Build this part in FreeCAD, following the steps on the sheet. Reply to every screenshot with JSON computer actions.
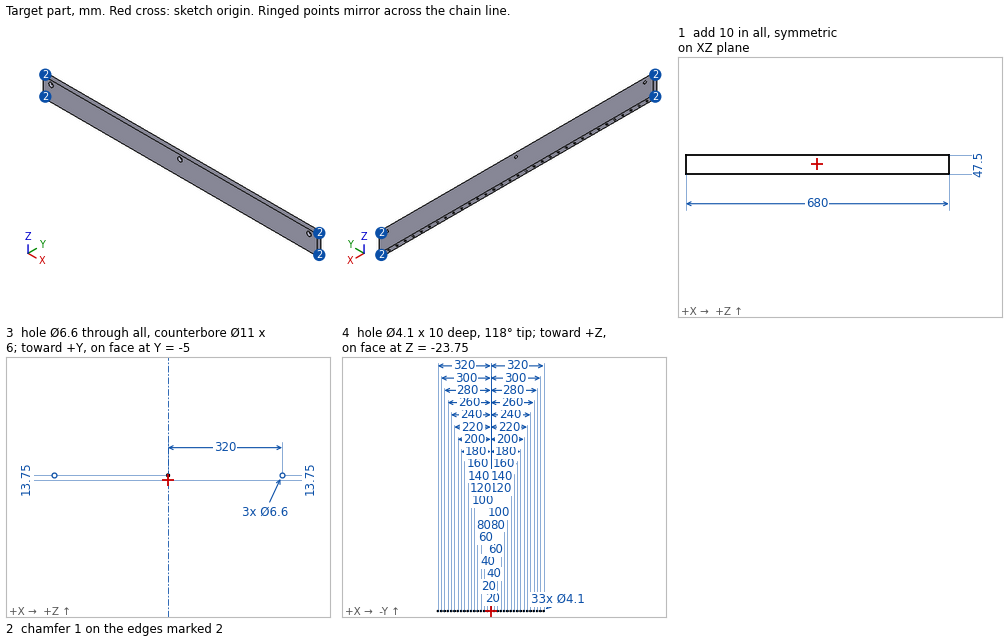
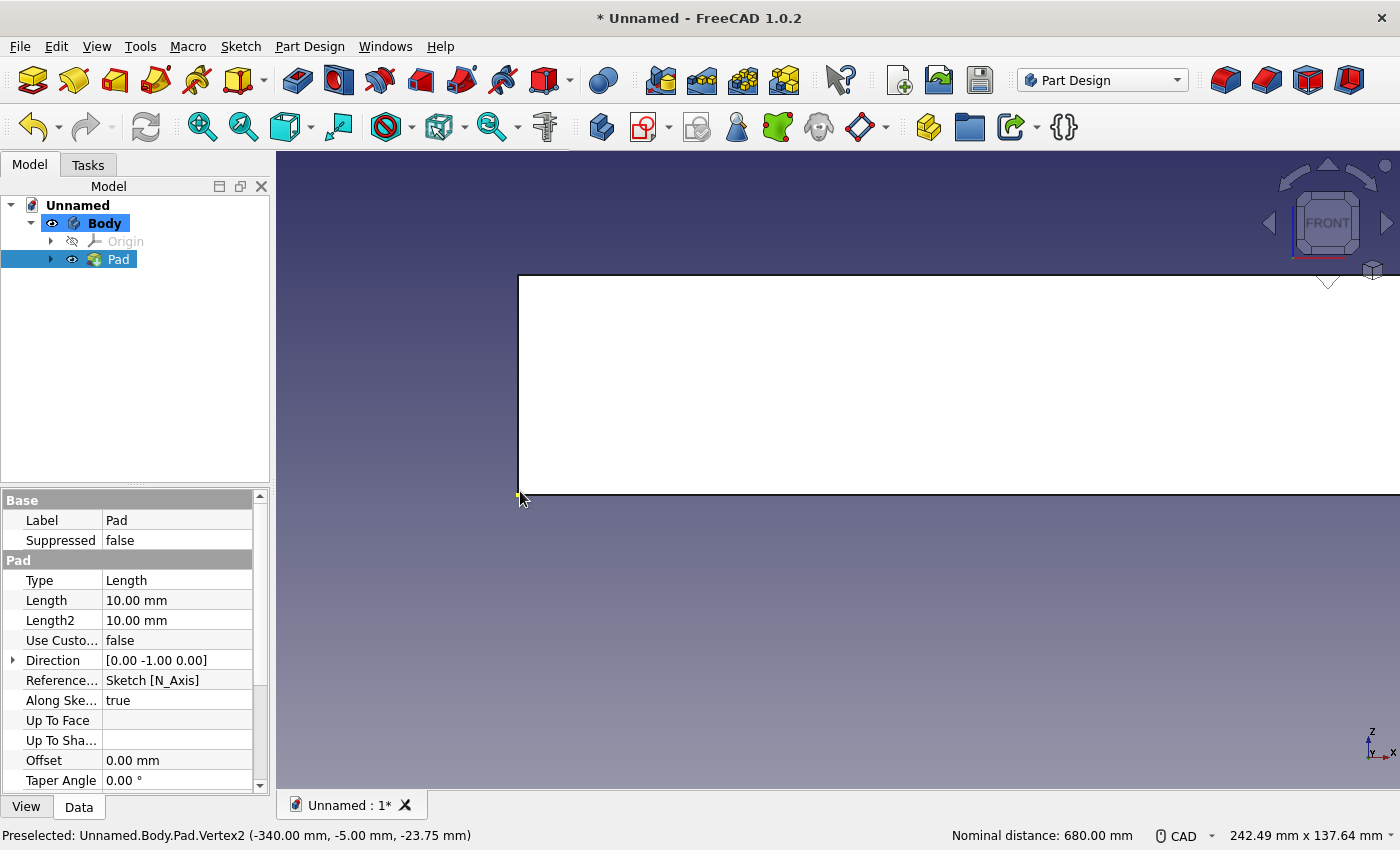
{"action": "left_click", "coordinate": [203, 128]}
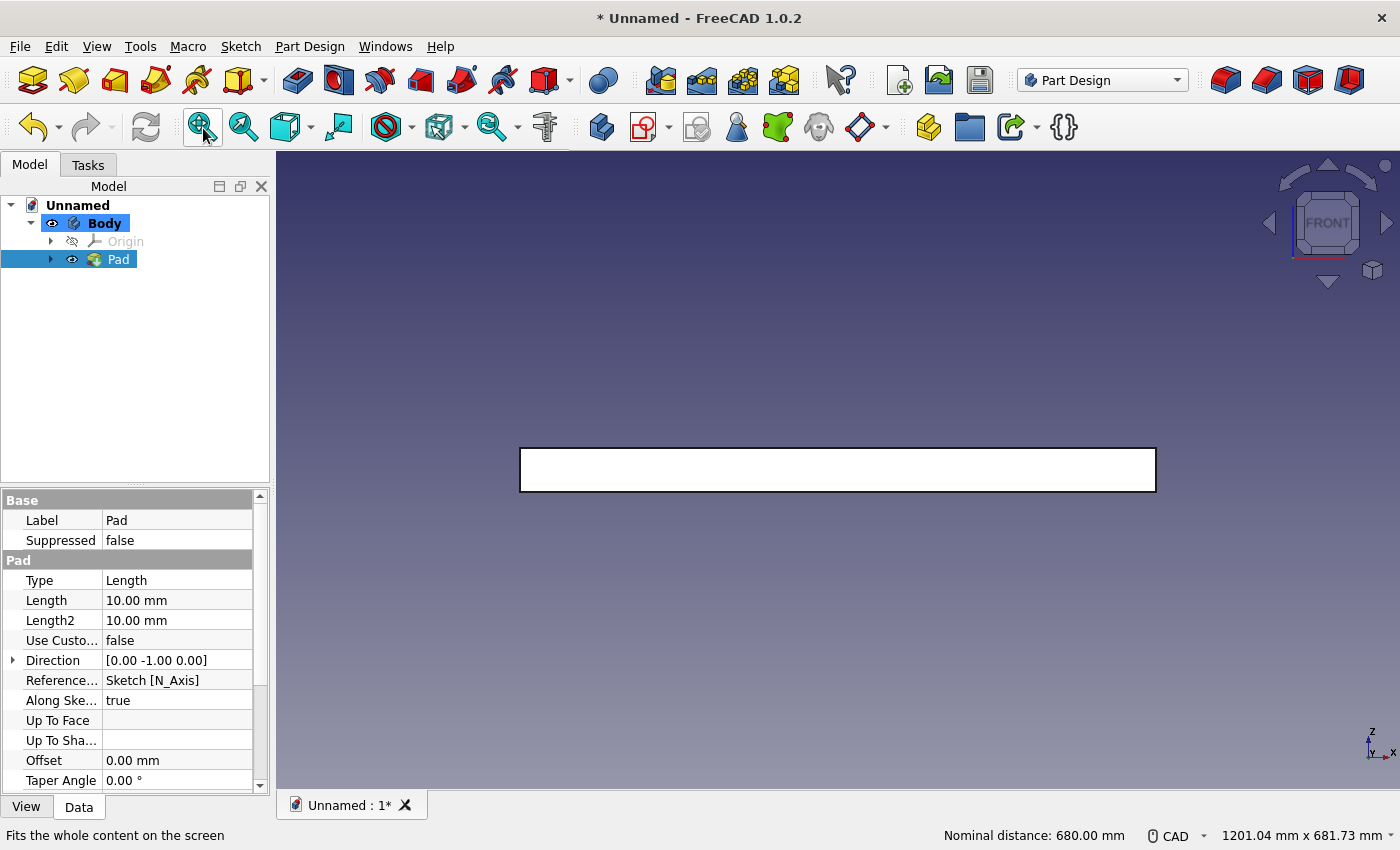
{"action": "key", "text": "3"}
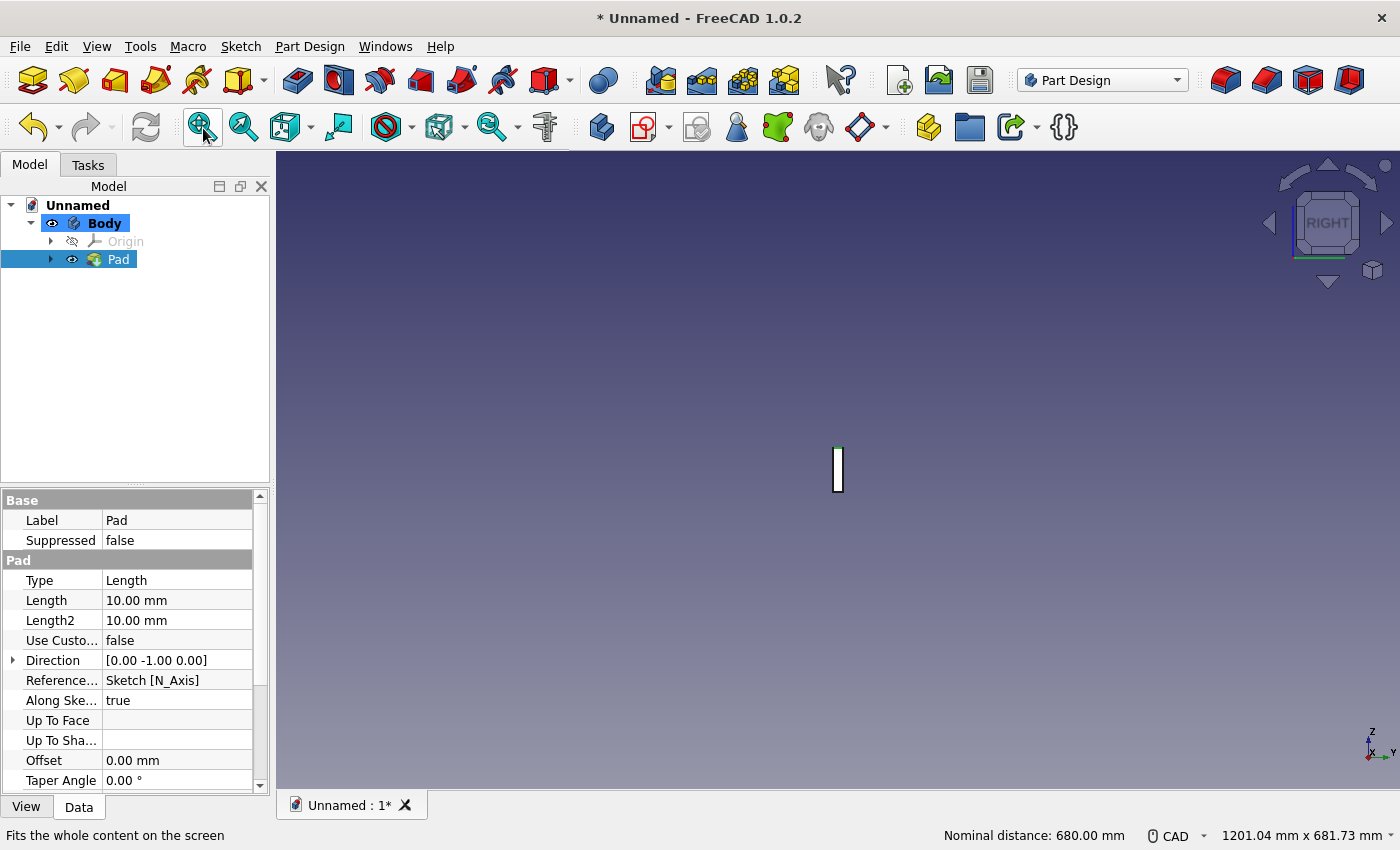
{"action": "left_click", "coordinate": [203, 128]}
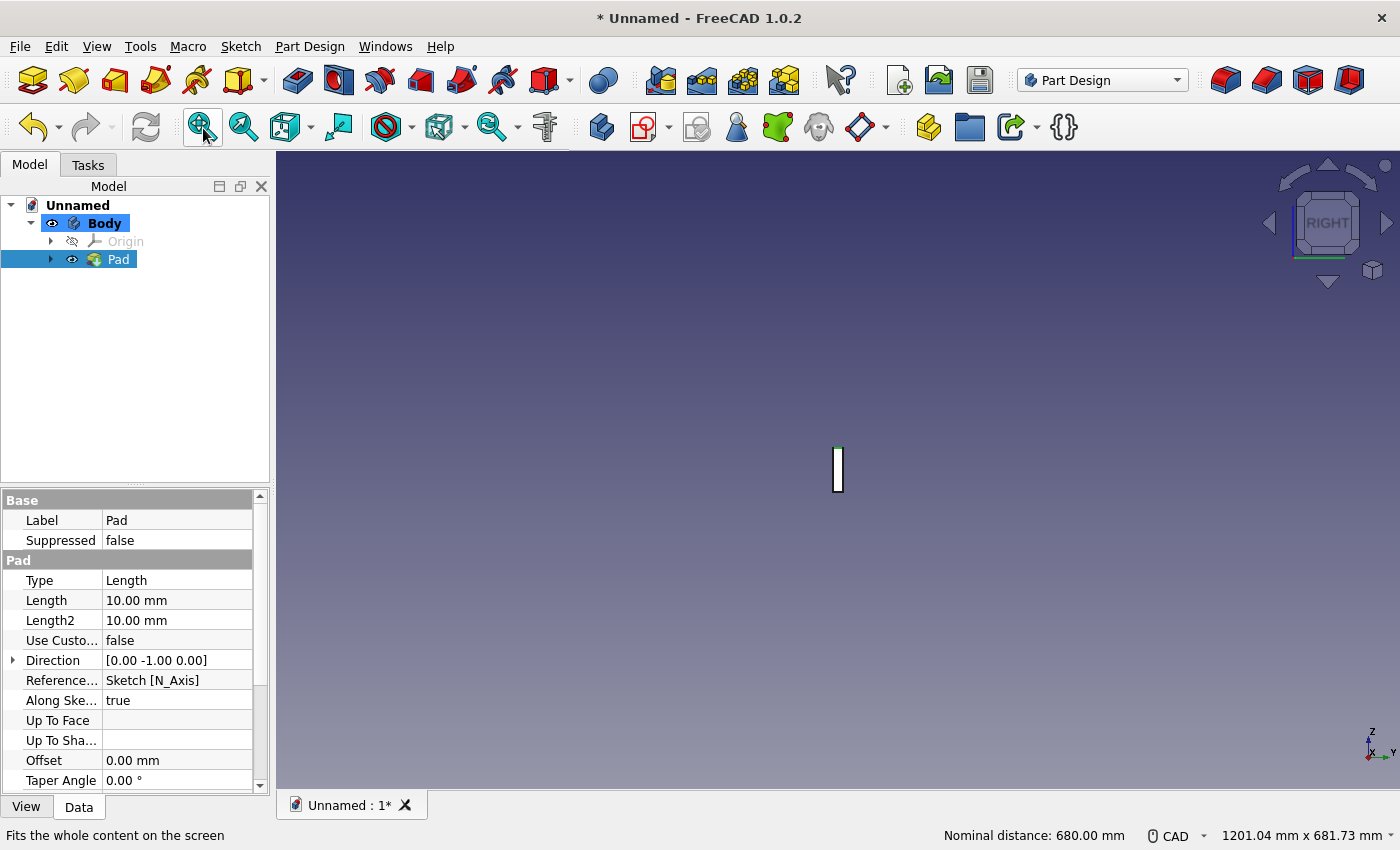
{"action": "scroll", "coordinate": [838, 491], "scroll_direction": "up", "scroll_amount": 8}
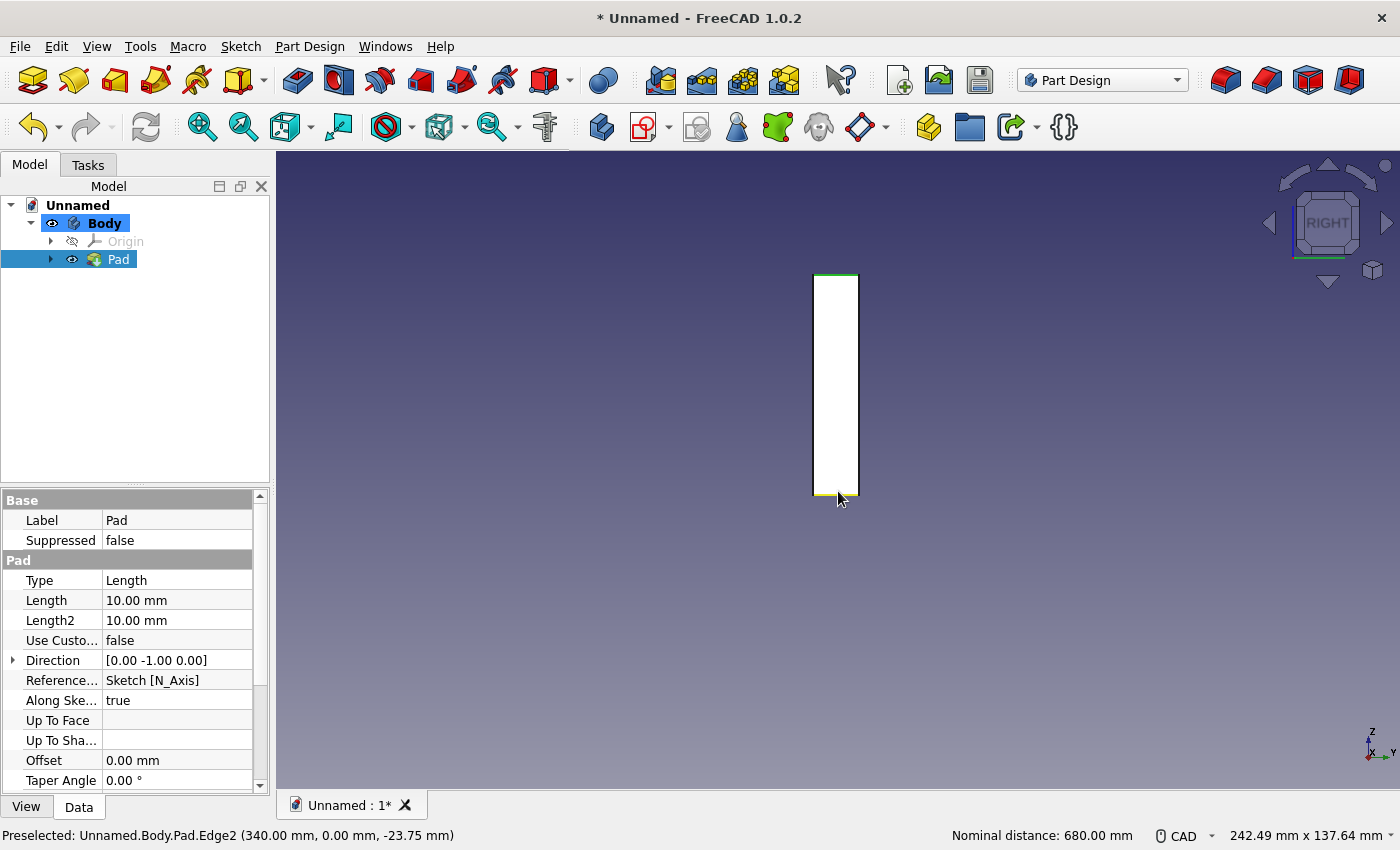
{"action": "left_click", "coordinate": [836, 494], "text": "ctrl"}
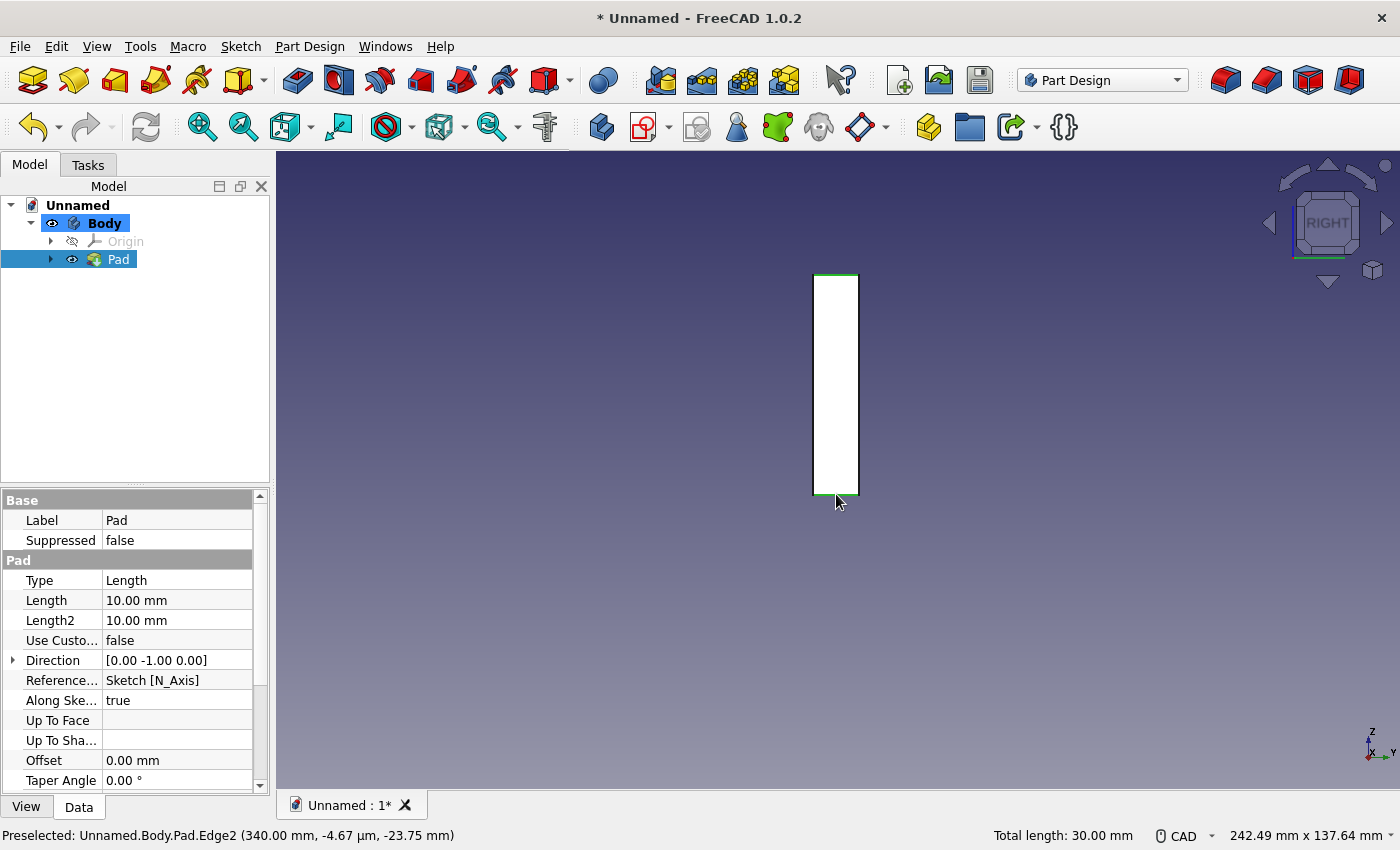
{"action": "left_click", "coordinate": [203, 128]}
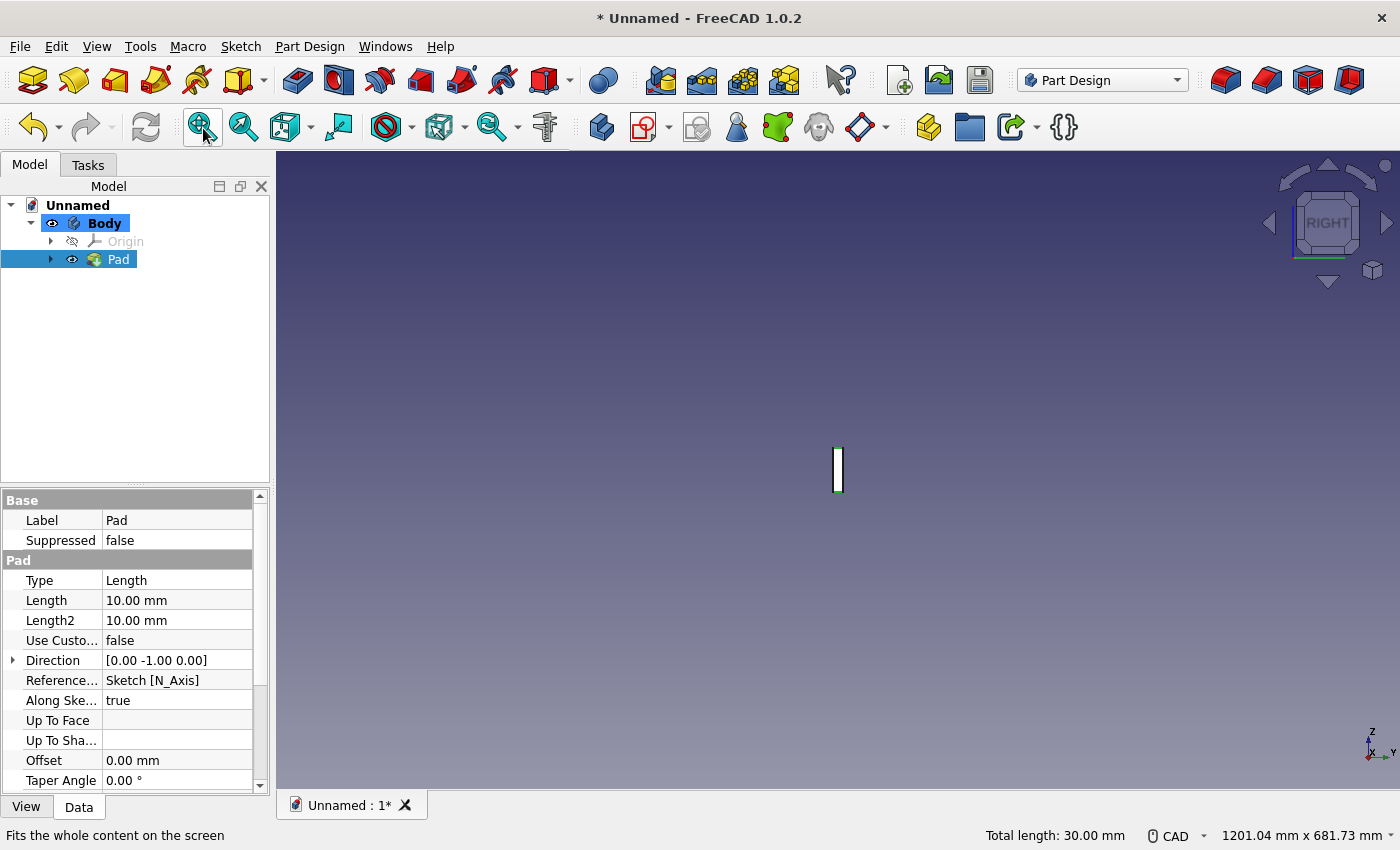
{"action": "key", "text": "5"}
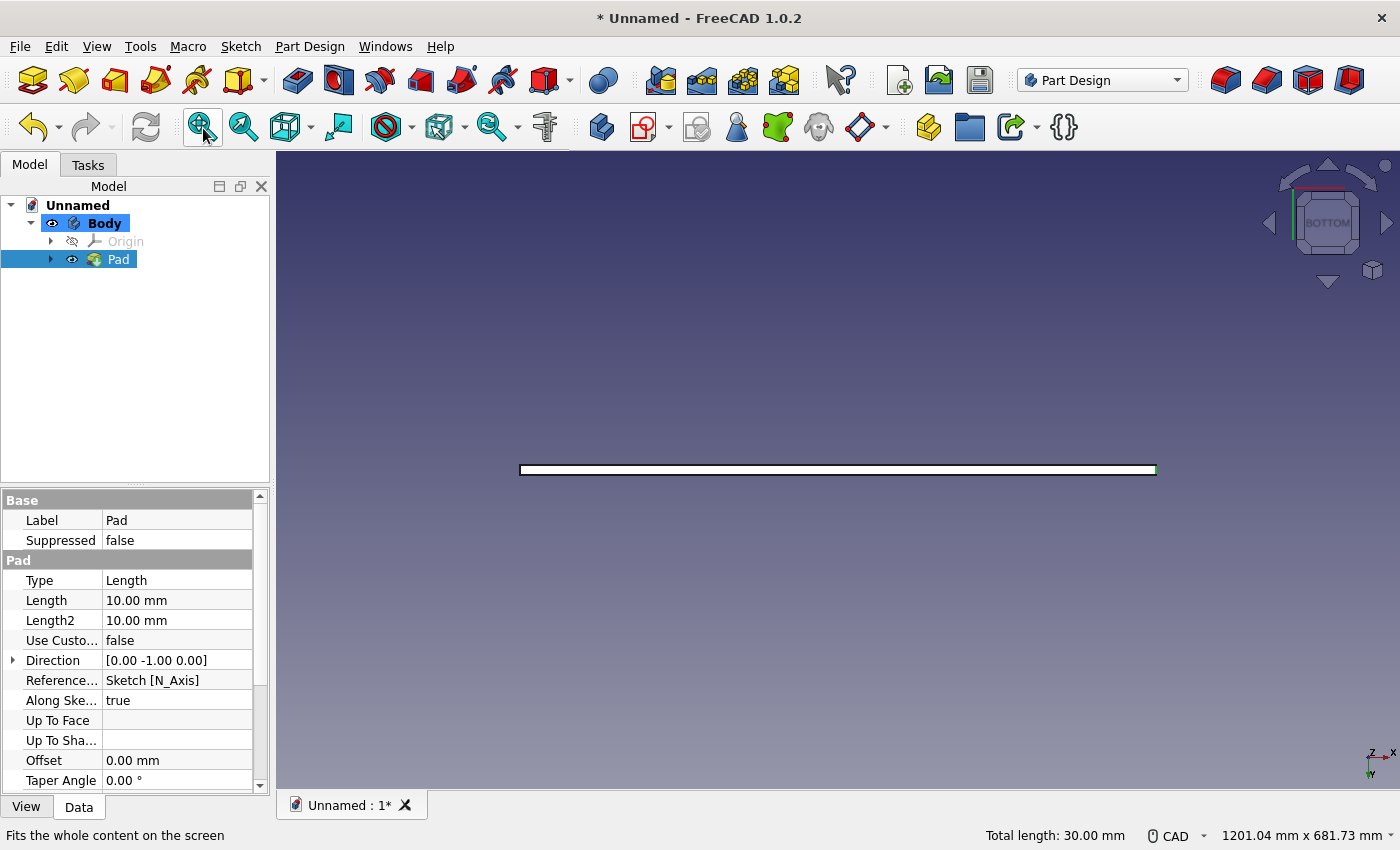
{"action": "left_click", "coordinate": [520, 471], "text": "ctrl"}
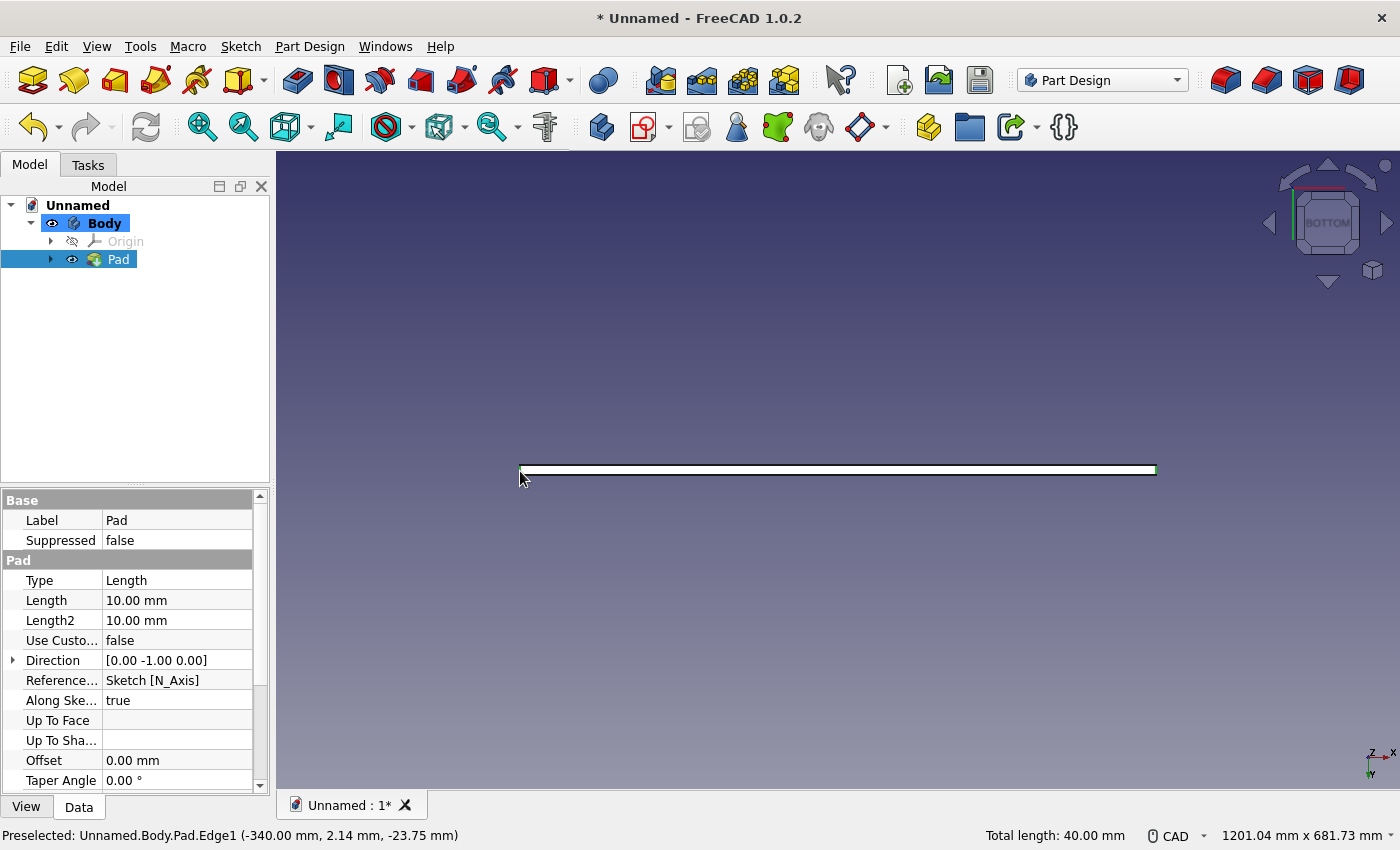
{"action": "left_click", "coordinate": [1267, 80]}